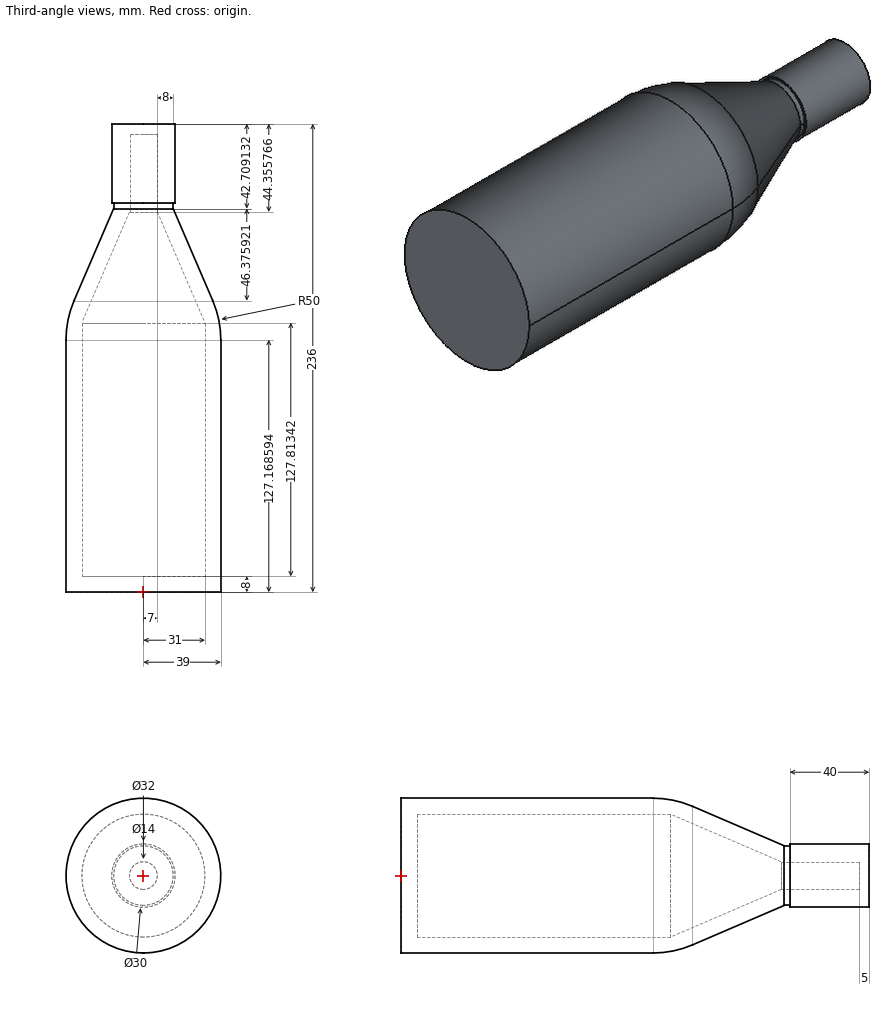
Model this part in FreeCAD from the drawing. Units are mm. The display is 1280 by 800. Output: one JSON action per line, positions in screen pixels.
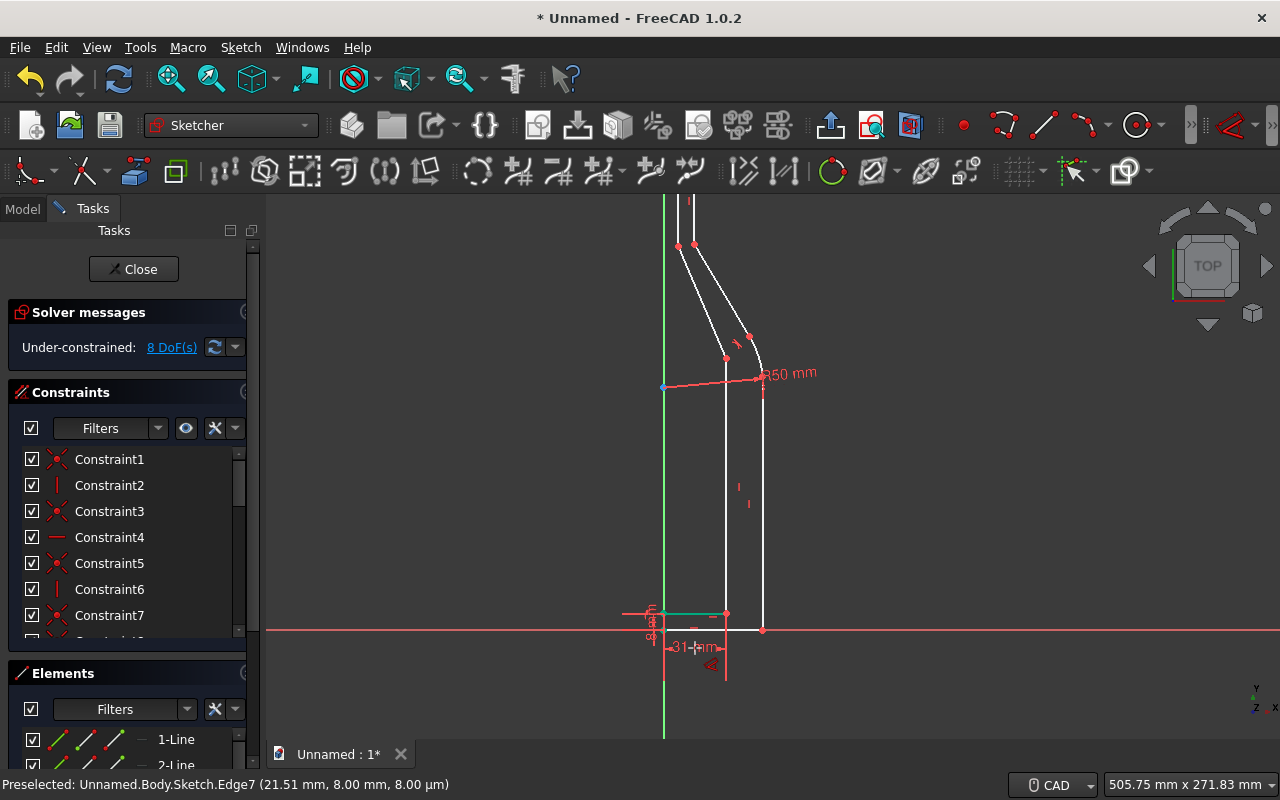
{"action": "left_click", "coordinate": [694, 630]}
{"action": "left_click", "coordinate": [691, 596]}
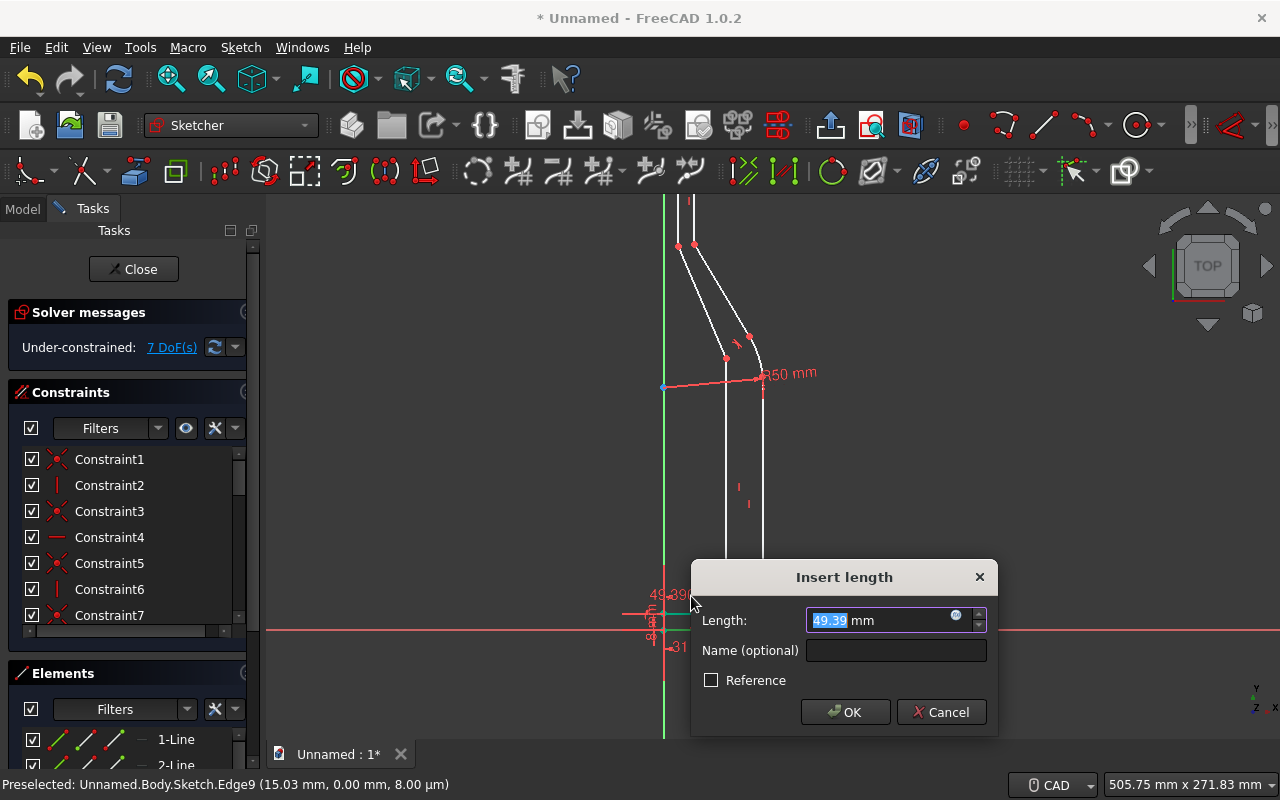
{"action": "type", "text": "39"}
{"action": "key", "text": "Return"}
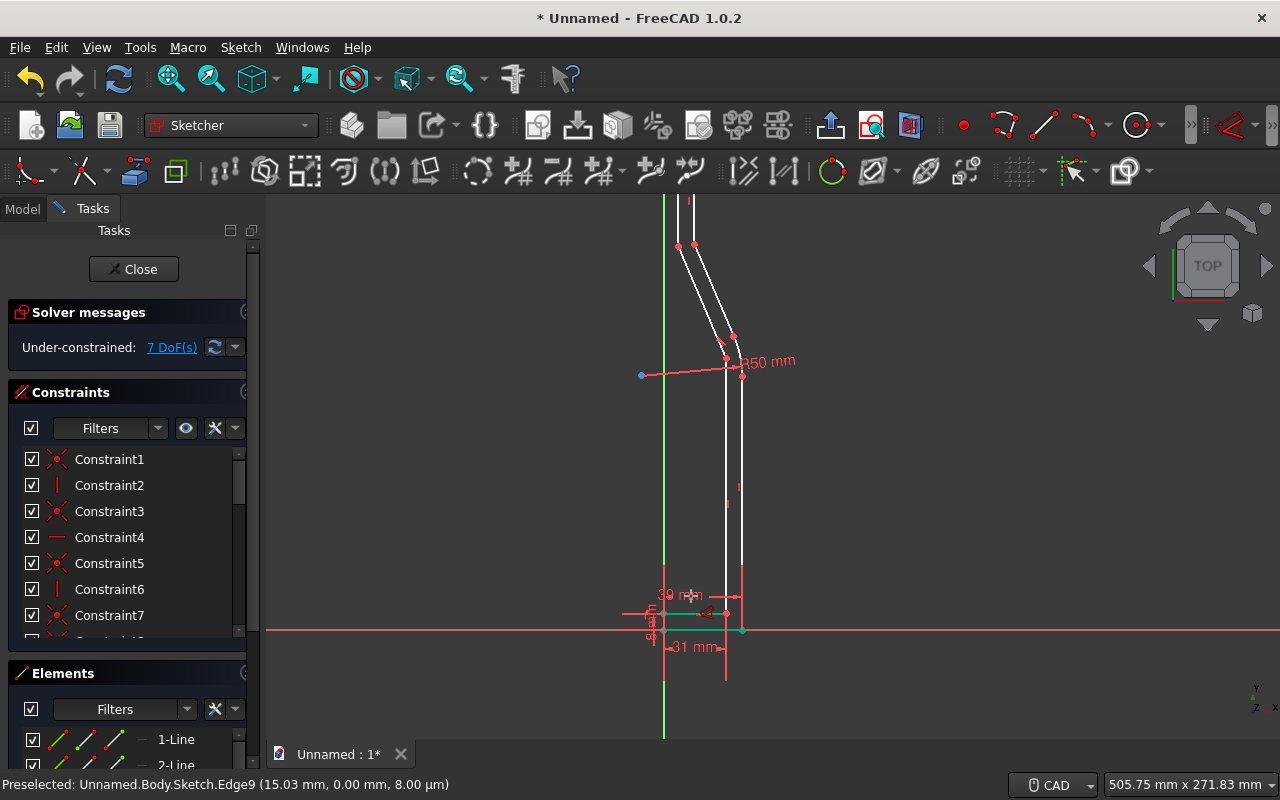
{"action": "scroll", "coordinate": [708, 615], "scroll_direction": "down", "scroll_amount": 2}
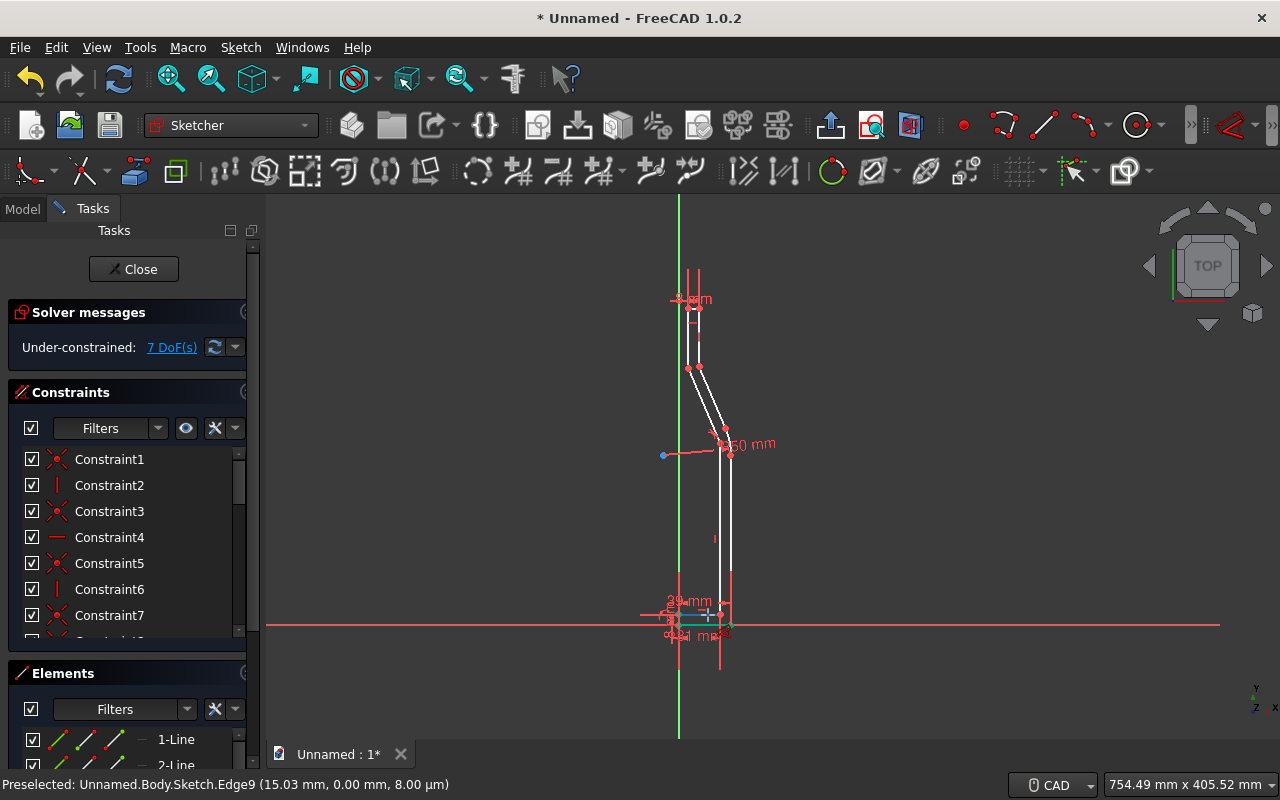
{"action": "scroll", "coordinate": [688, 309], "scroll_direction": "up", "scroll_amount": 8}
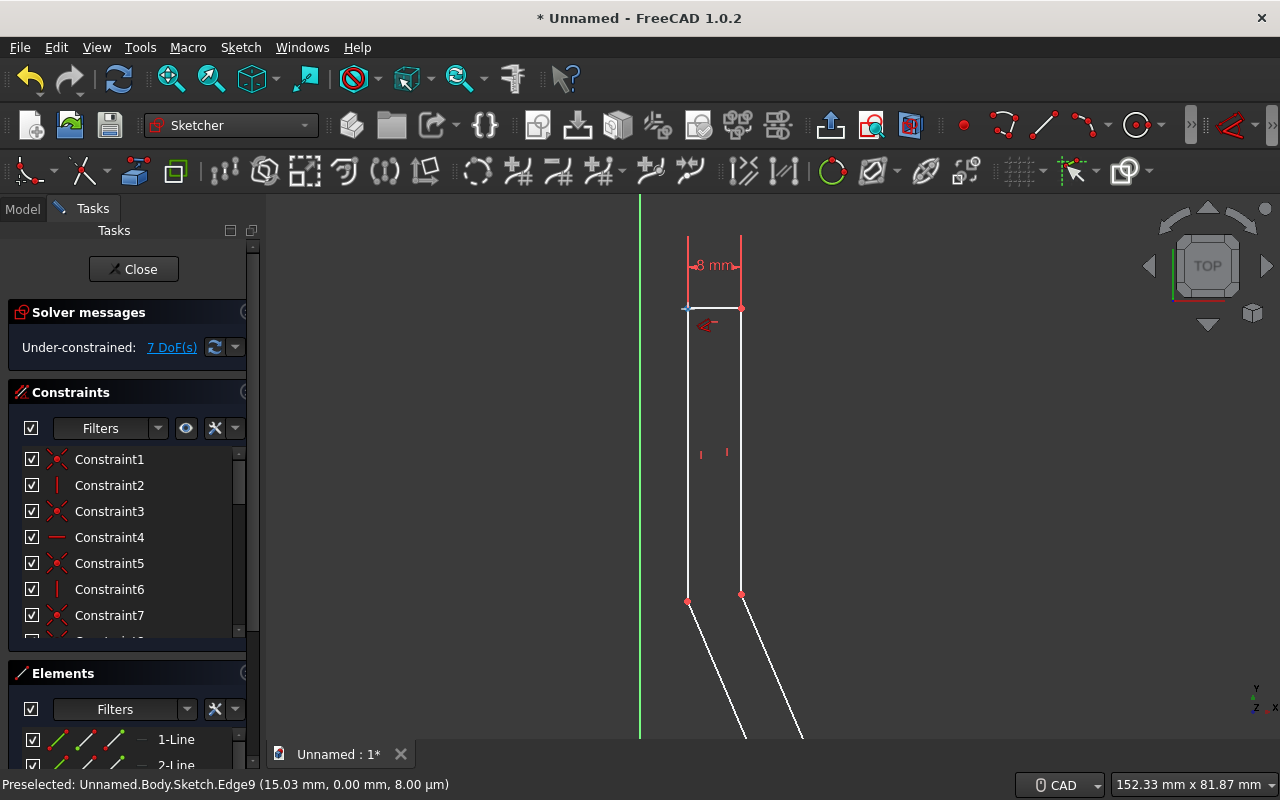
{"action": "left_click", "coordinate": [688, 308]}
{"action": "left_click", "coordinate": [664, 226]}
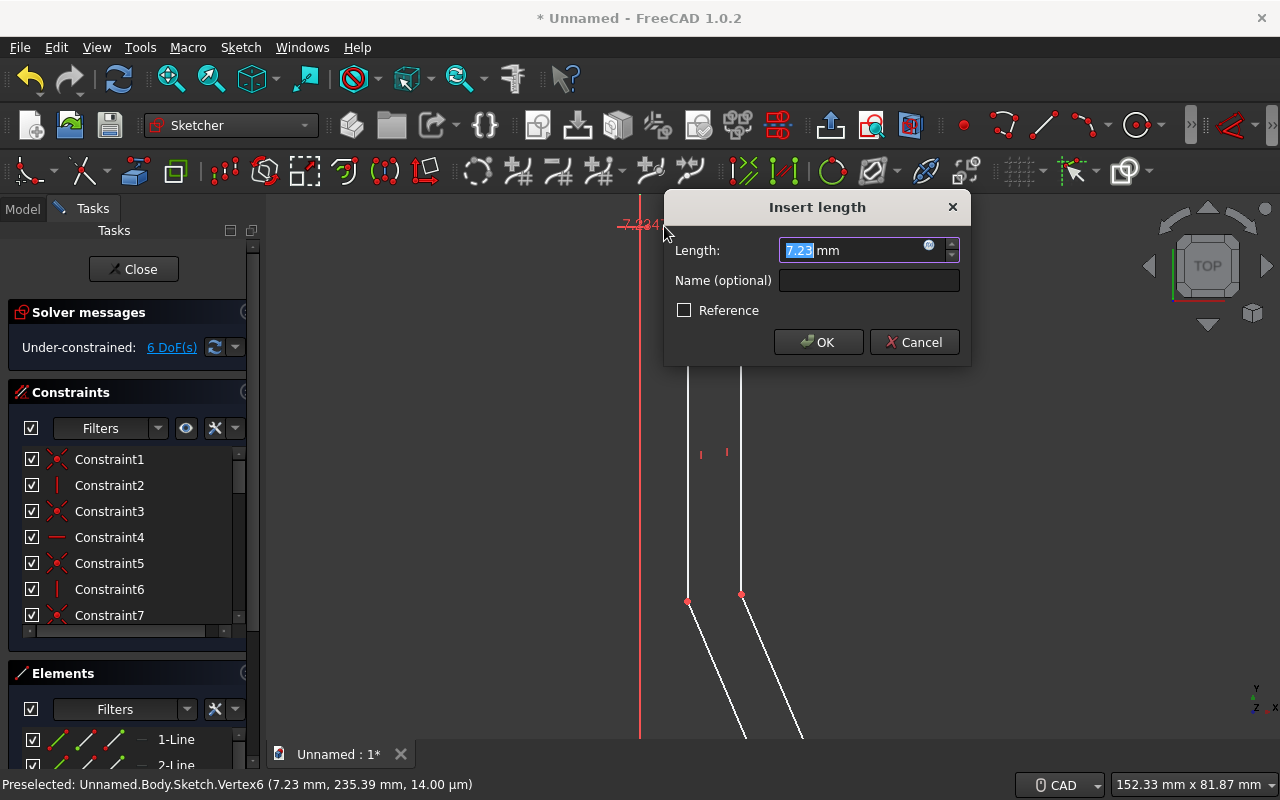
{"action": "type", "text": "7"}
{"action": "key", "text": "Return"}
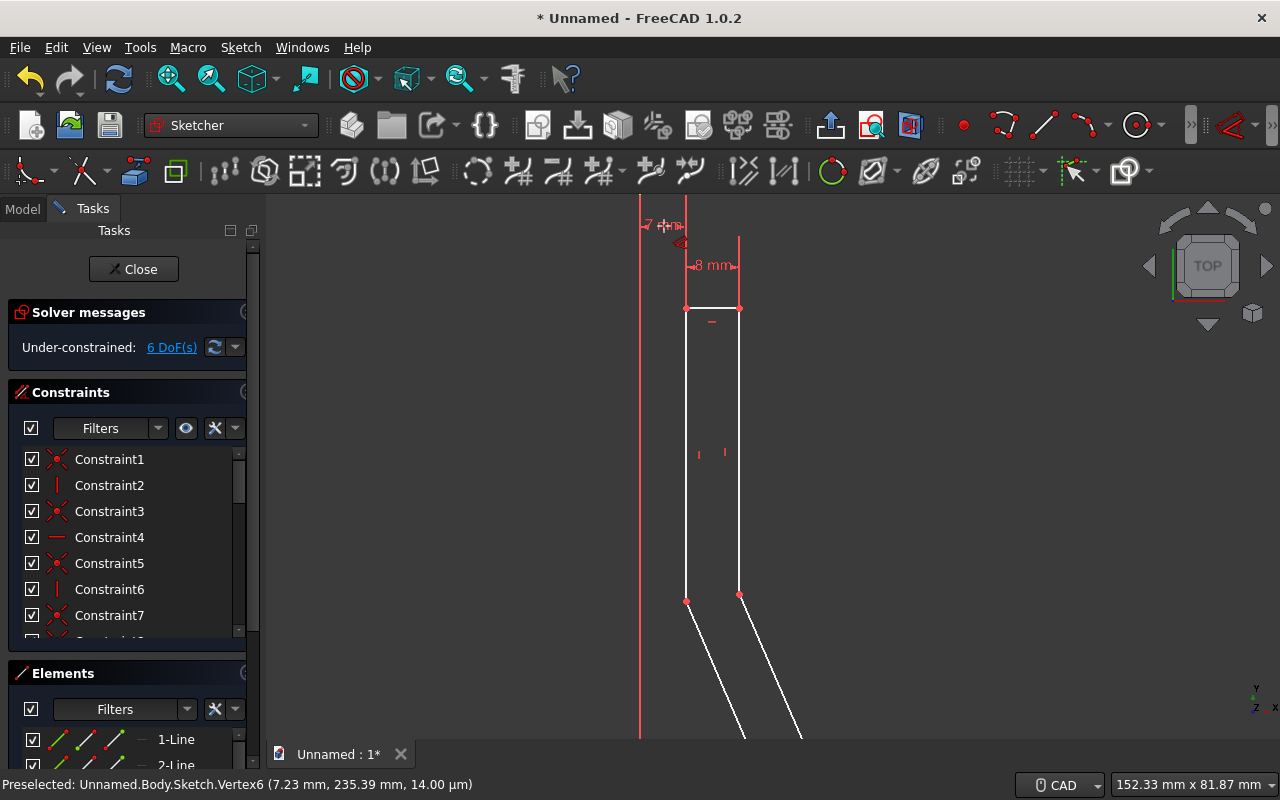
{"action": "scroll", "coordinate": [688, 309], "scroll_direction": "down", "scroll_amount": 8}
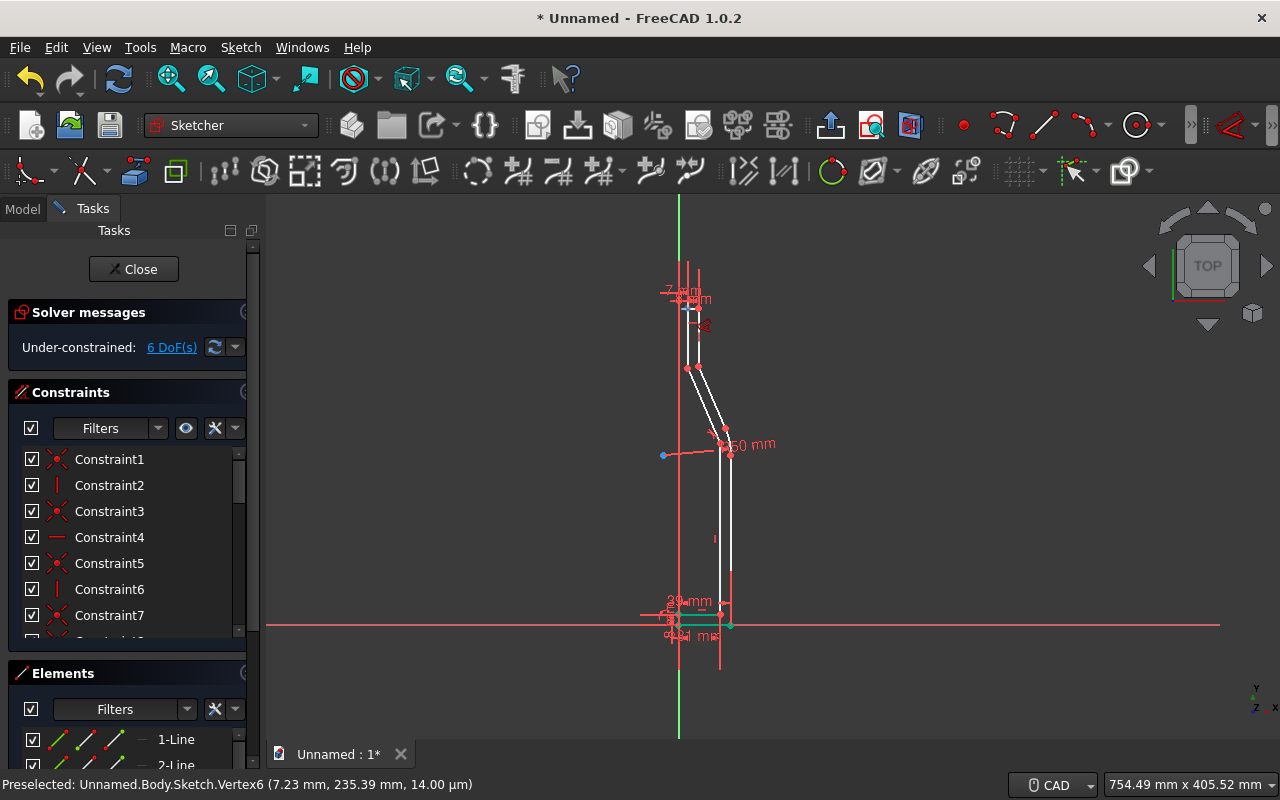
{"action": "left_click", "coordinate": [699, 309]}
{"action": "left_click", "coordinate": [645, 467]}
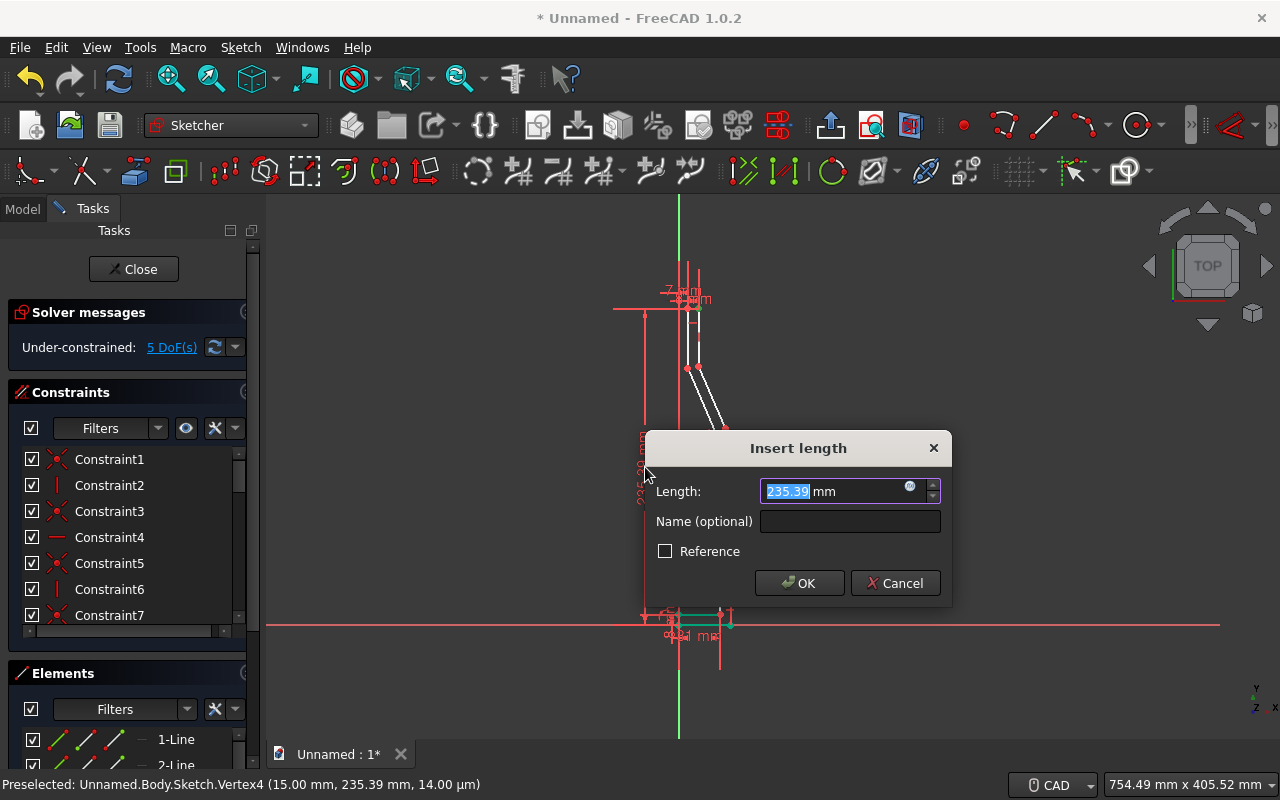
{"action": "type", "text": "236"}
{"action": "key", "text": "Return"}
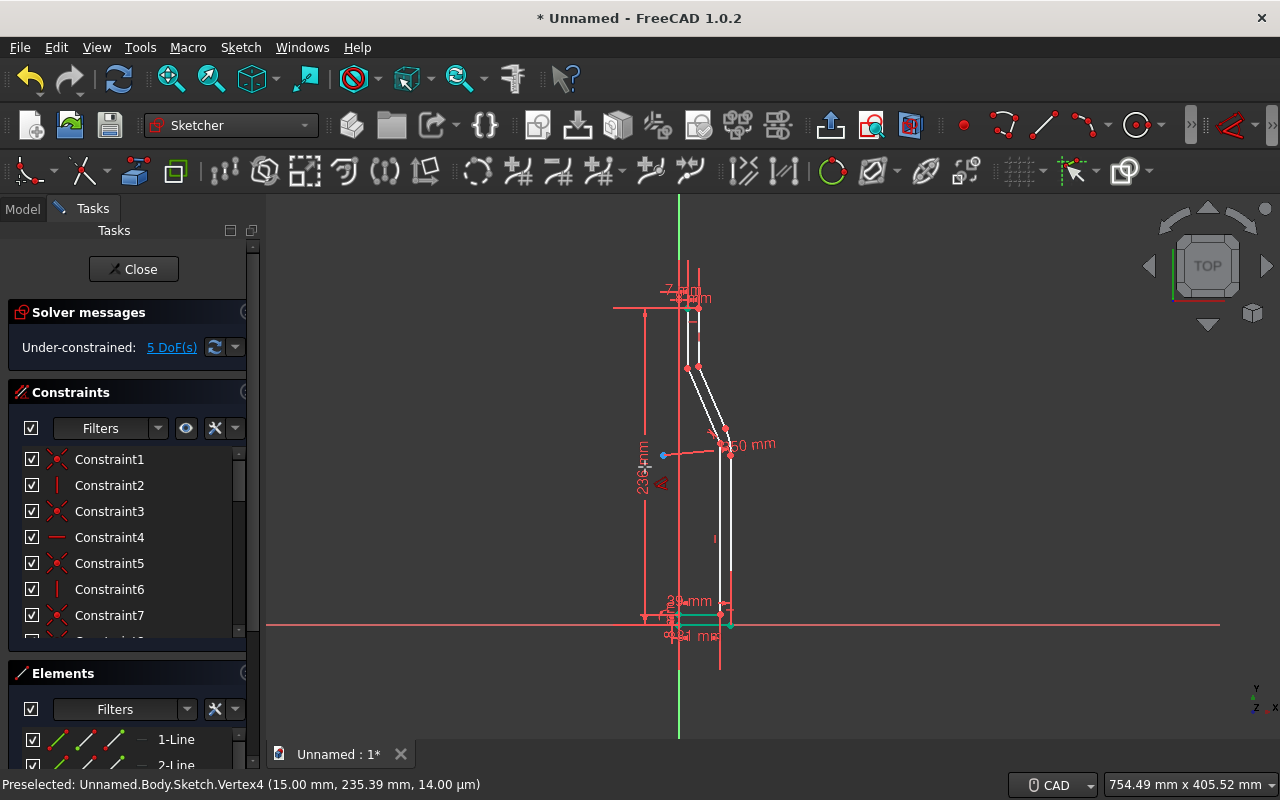
{"action": "scroll", "coordinate": [699, 349], "scroll_direction": "up", "scroll_amount": 2}